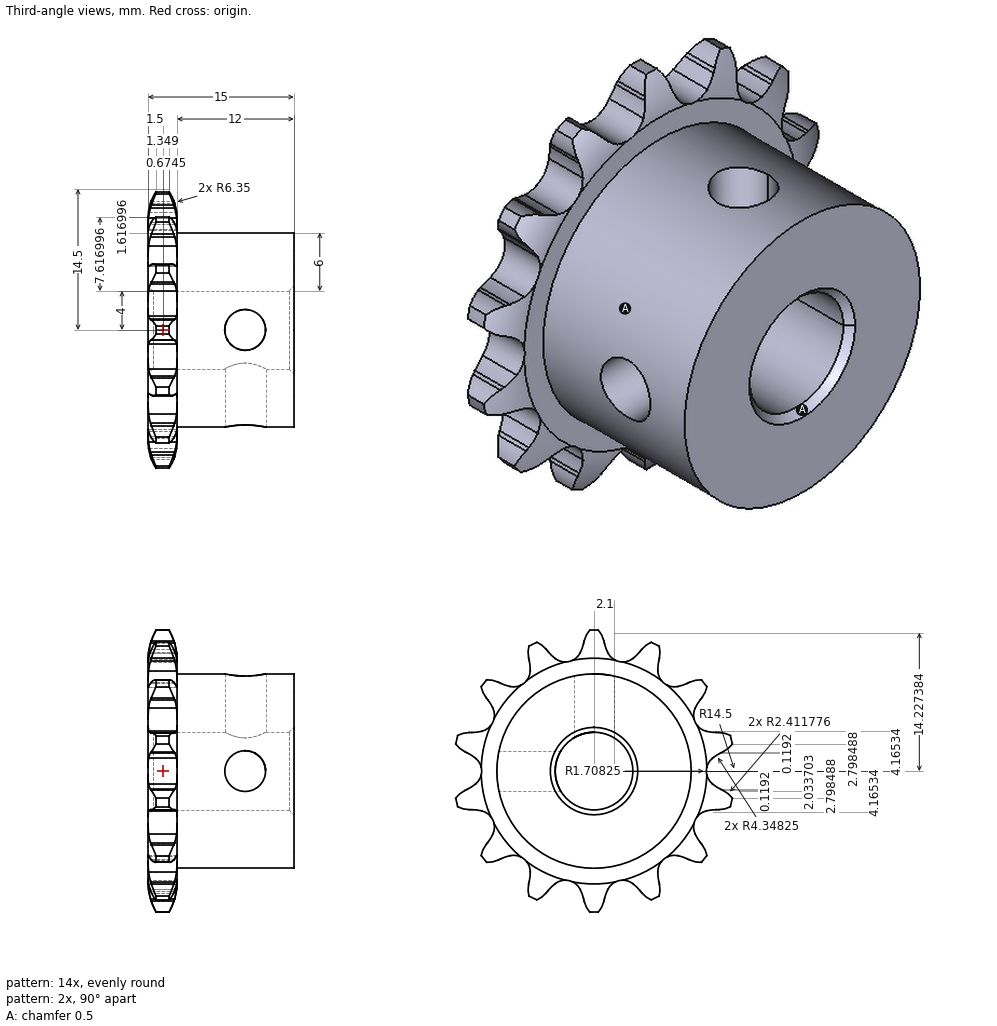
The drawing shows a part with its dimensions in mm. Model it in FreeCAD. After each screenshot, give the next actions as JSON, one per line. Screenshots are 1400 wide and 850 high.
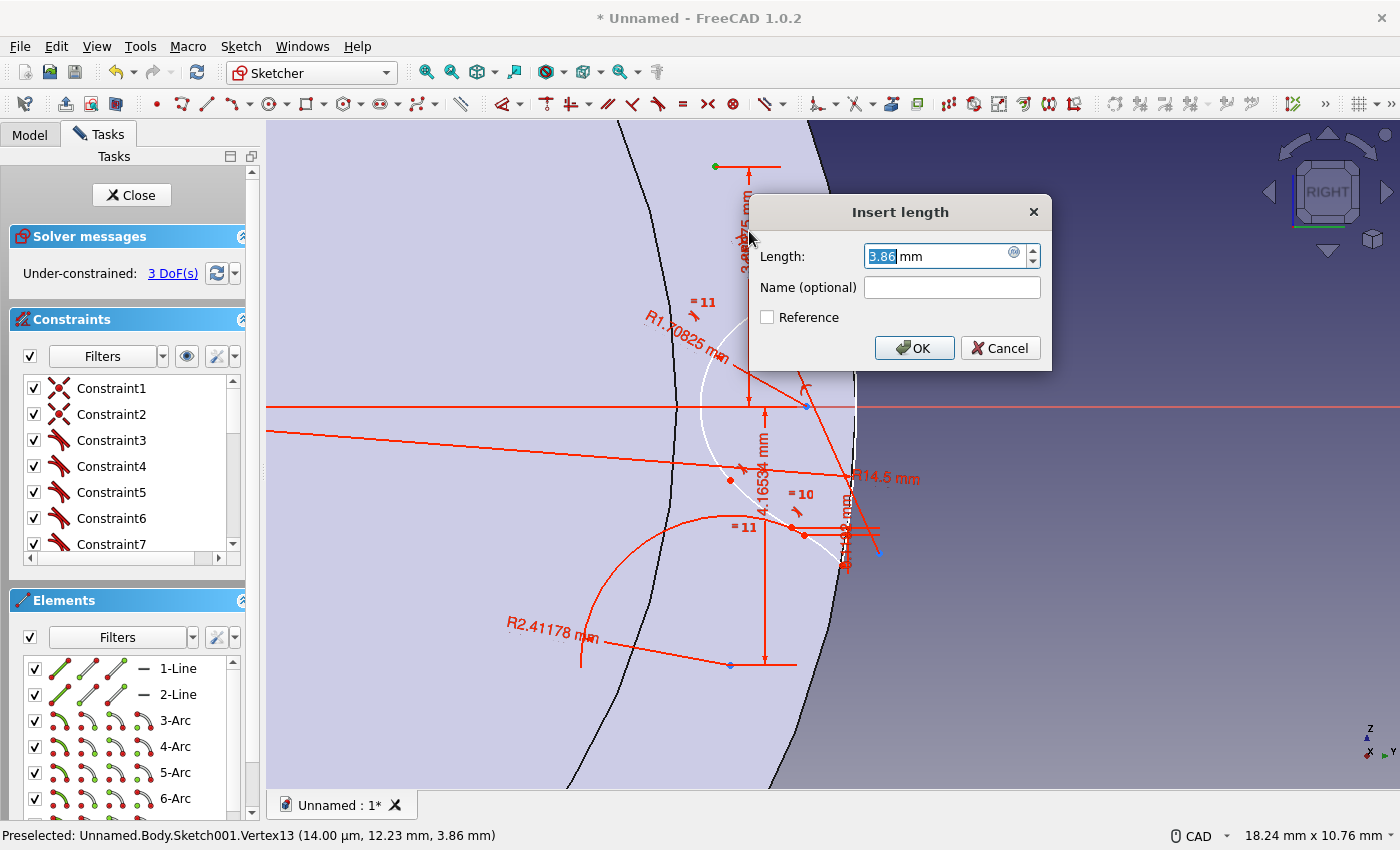
{"action": "type", "text": "4.16534"}
{"action": "key", "text": "Return"}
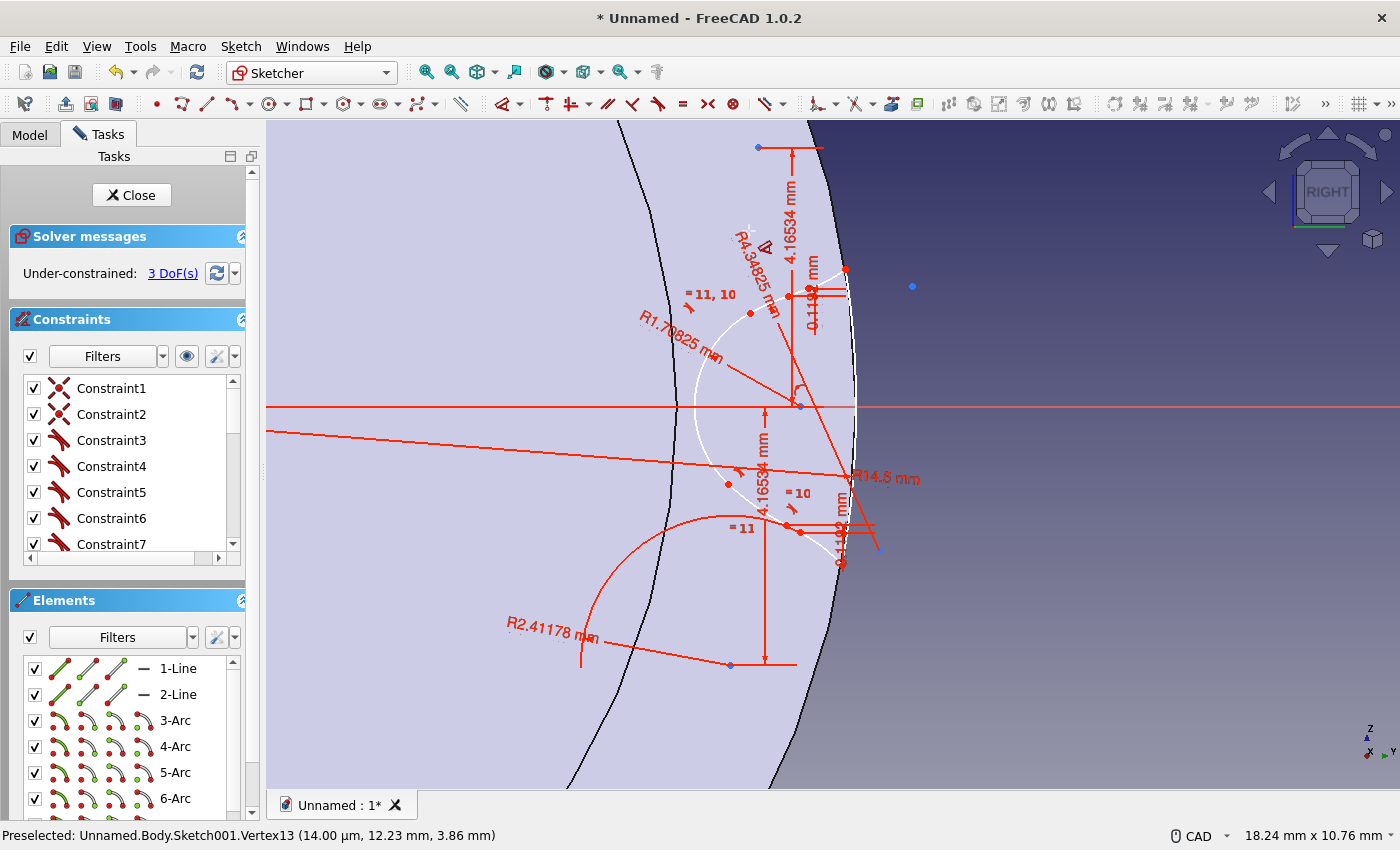
{"action": "left_click", "coordinate": [842, 565]}
{"action": "left_click", "coordinate": [876, 449]}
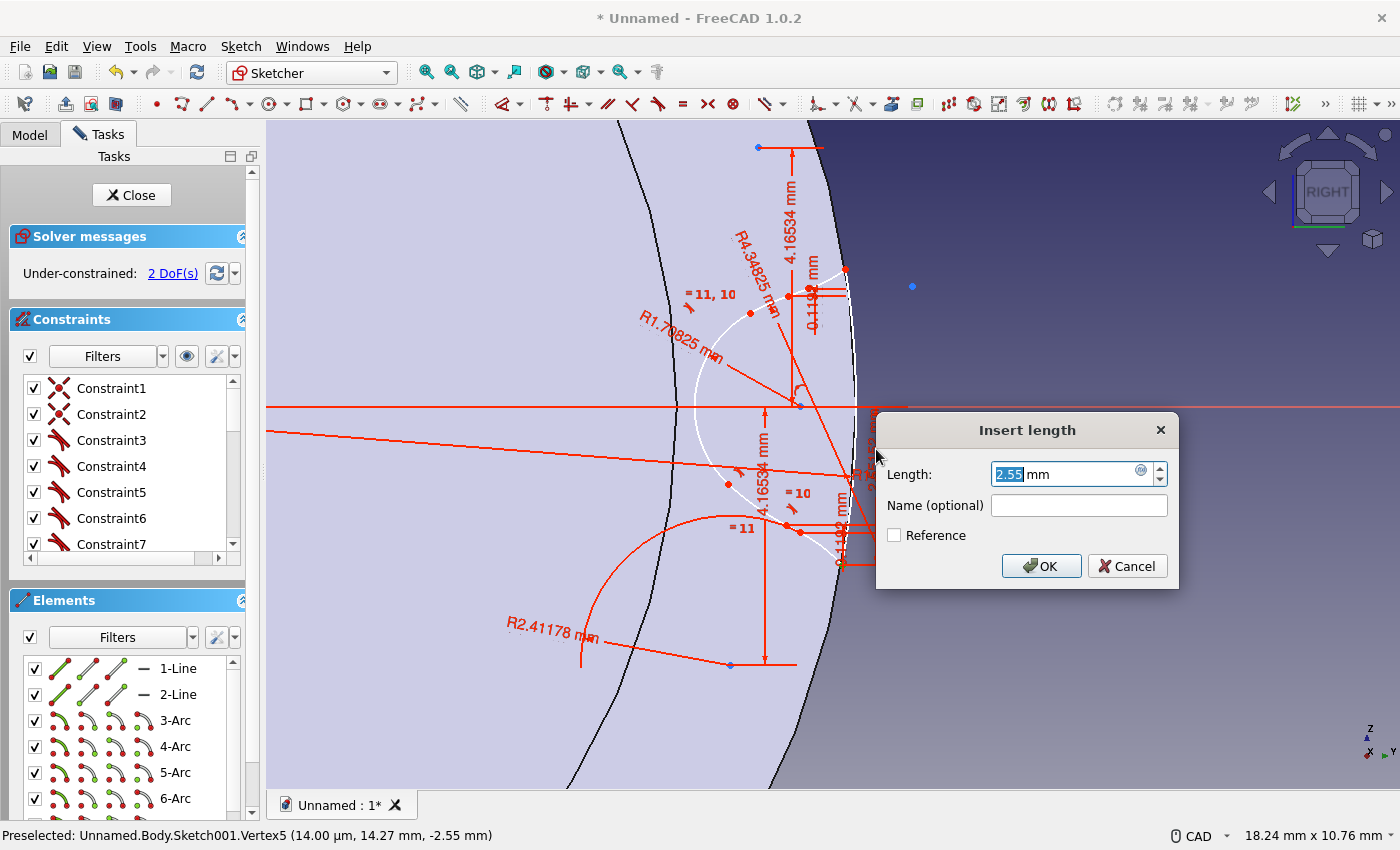
{"action": "type", "text": "2.798488"}
{"action": "key", "text": "Return"}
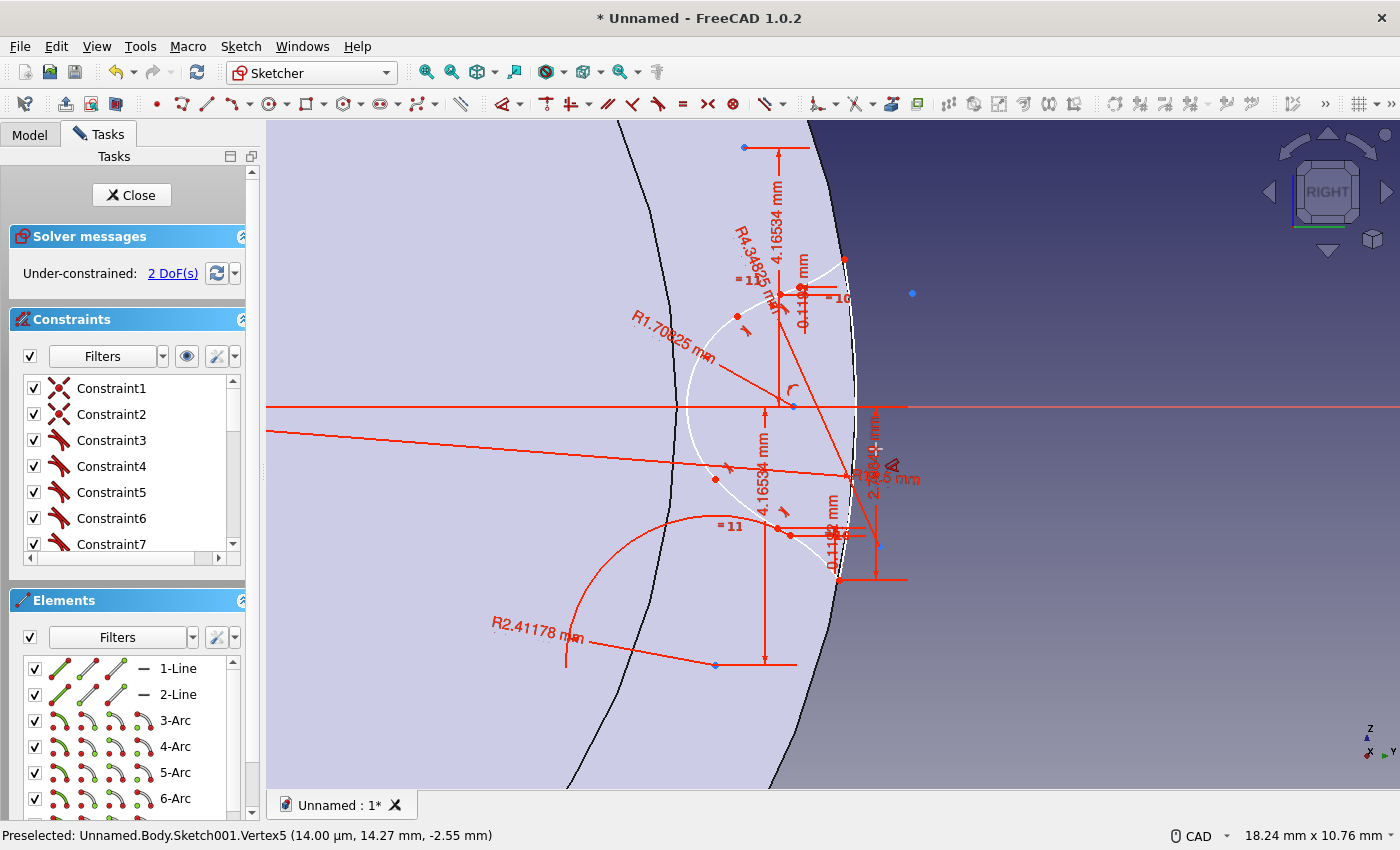
{"action": "left_click", "coordinate": [844, 260]}
{"action": "left_click", "coordinate": [878, 333]}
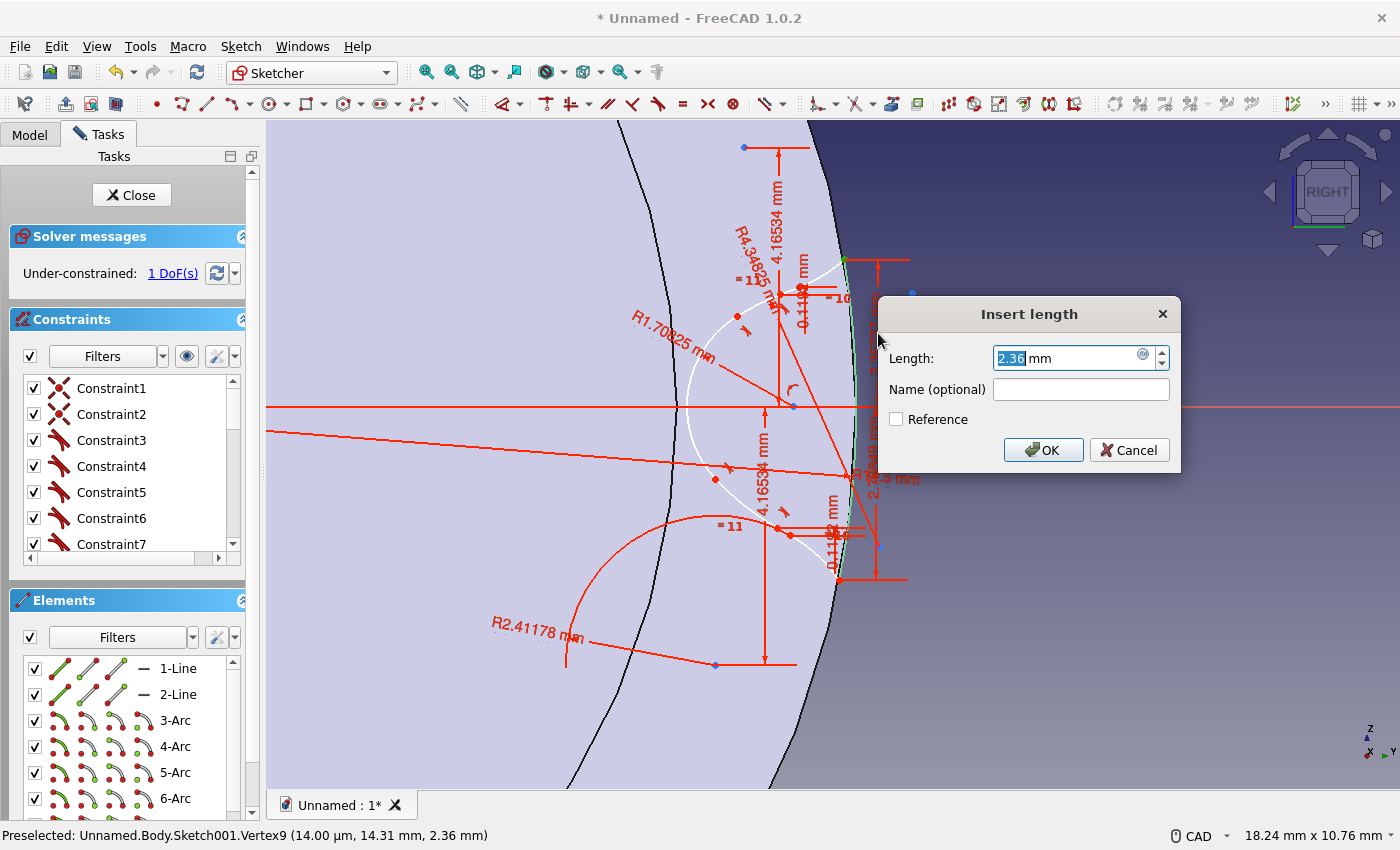
{"action": "type", "text": "2.798488"}
{"action": "key", "text": "Return"}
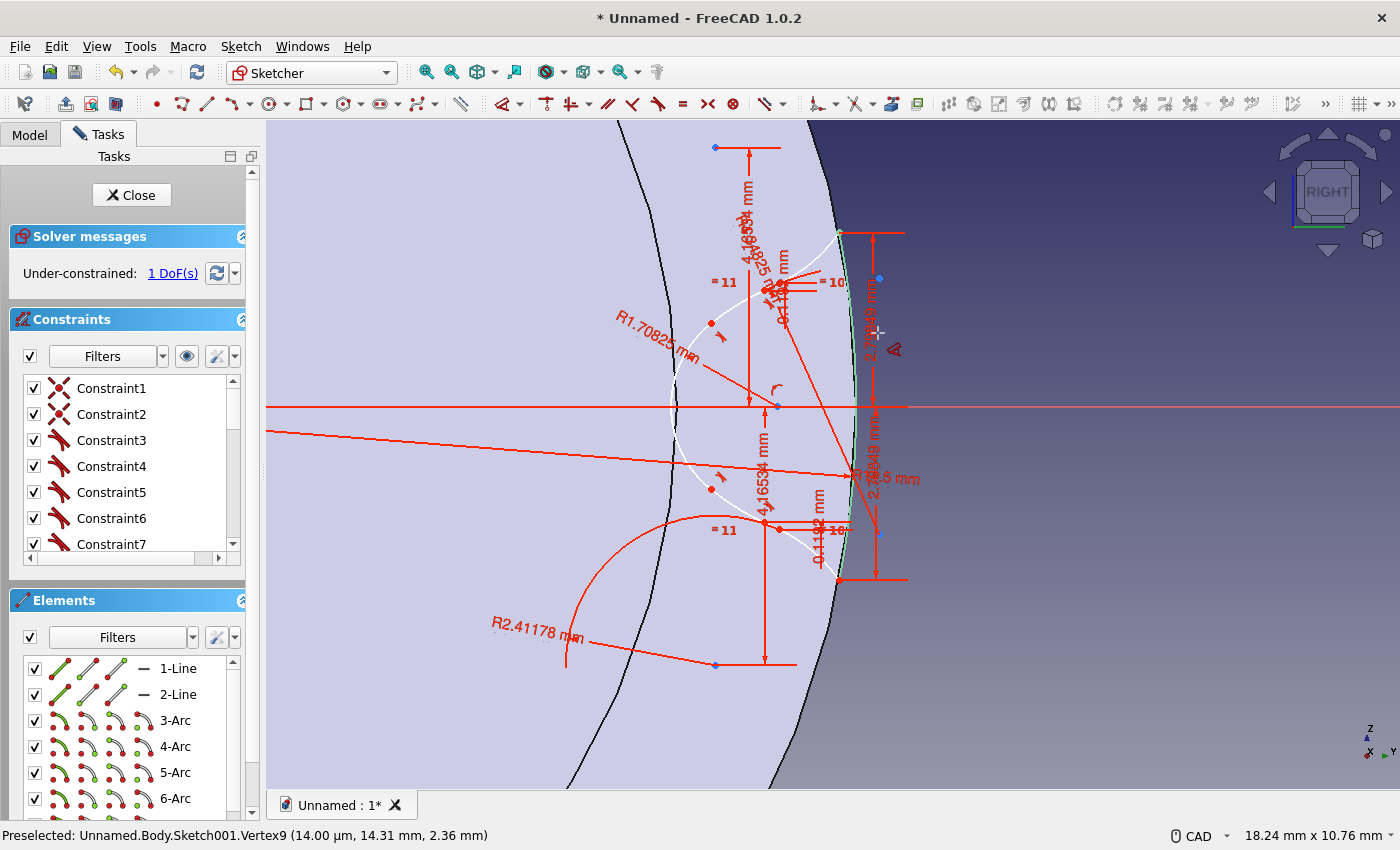
{"action": "left_click", "coordinate": [880, 535]}
{"action": "left_click", "coordinate": [914, 500]}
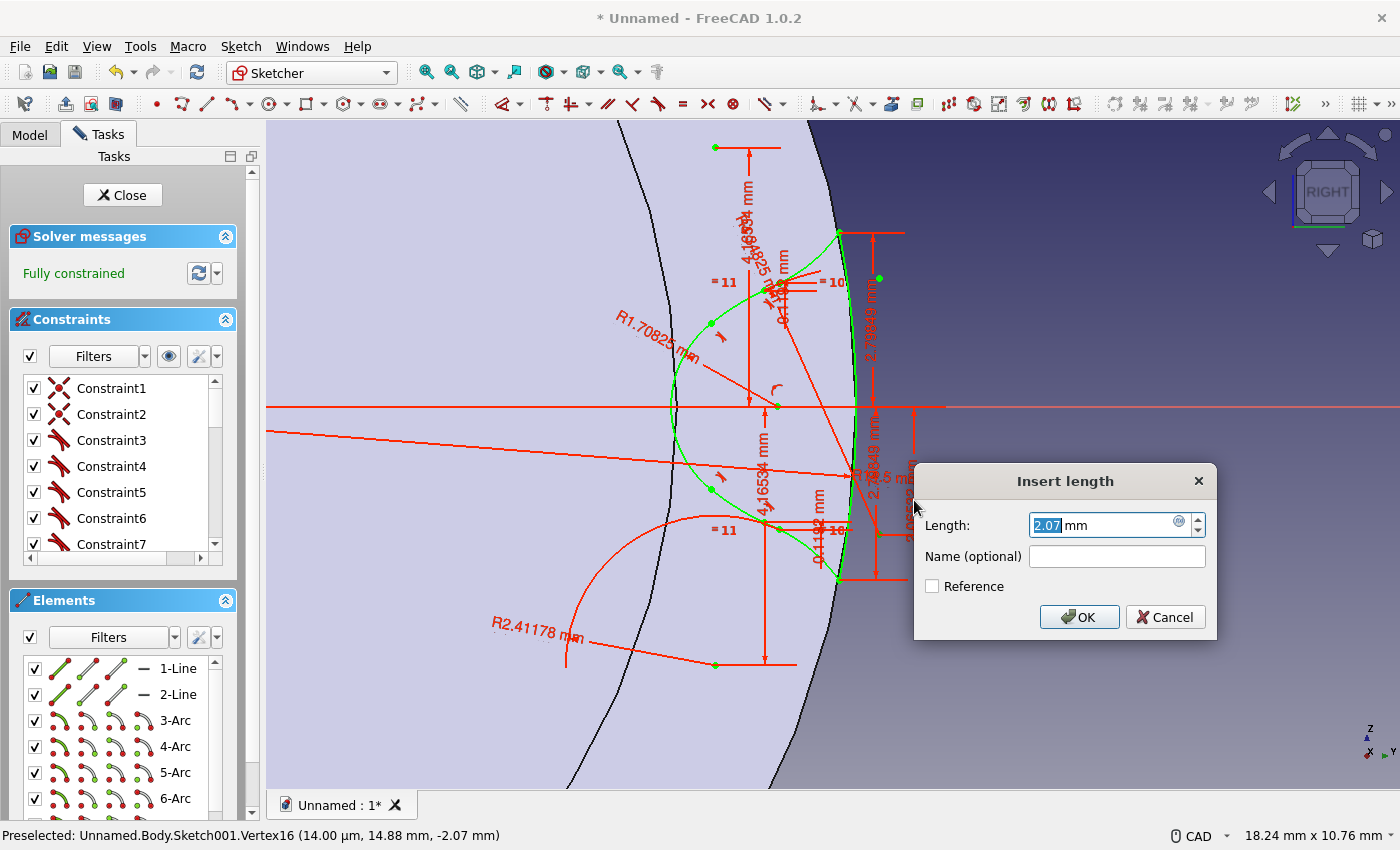
{"action": "type", "text": "2.033703"}
{"action": "key", "text": "Return"}
{"action": "key", "text": "Escape"}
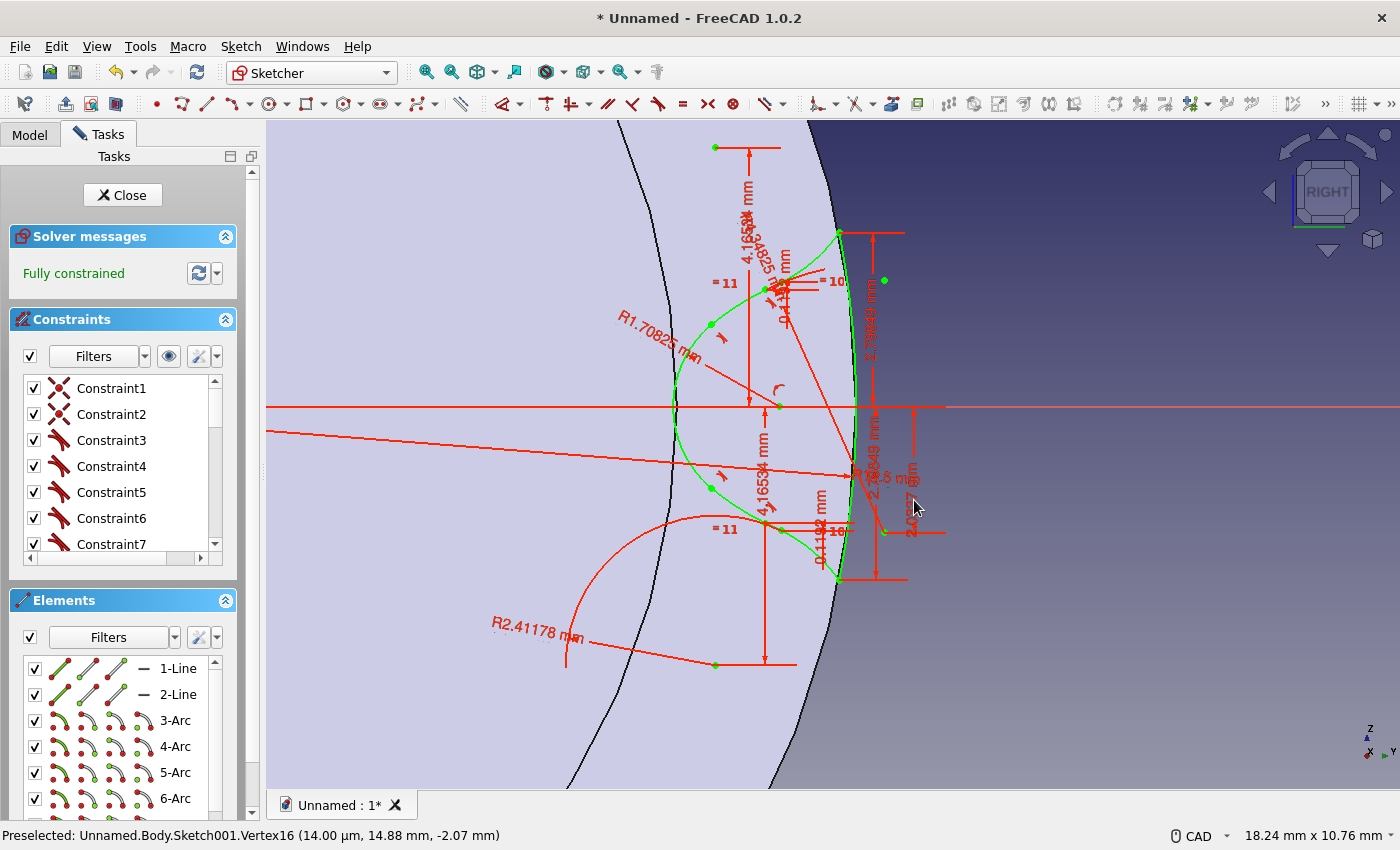
{"action": "left_click", "coordinate": [123, 195]}